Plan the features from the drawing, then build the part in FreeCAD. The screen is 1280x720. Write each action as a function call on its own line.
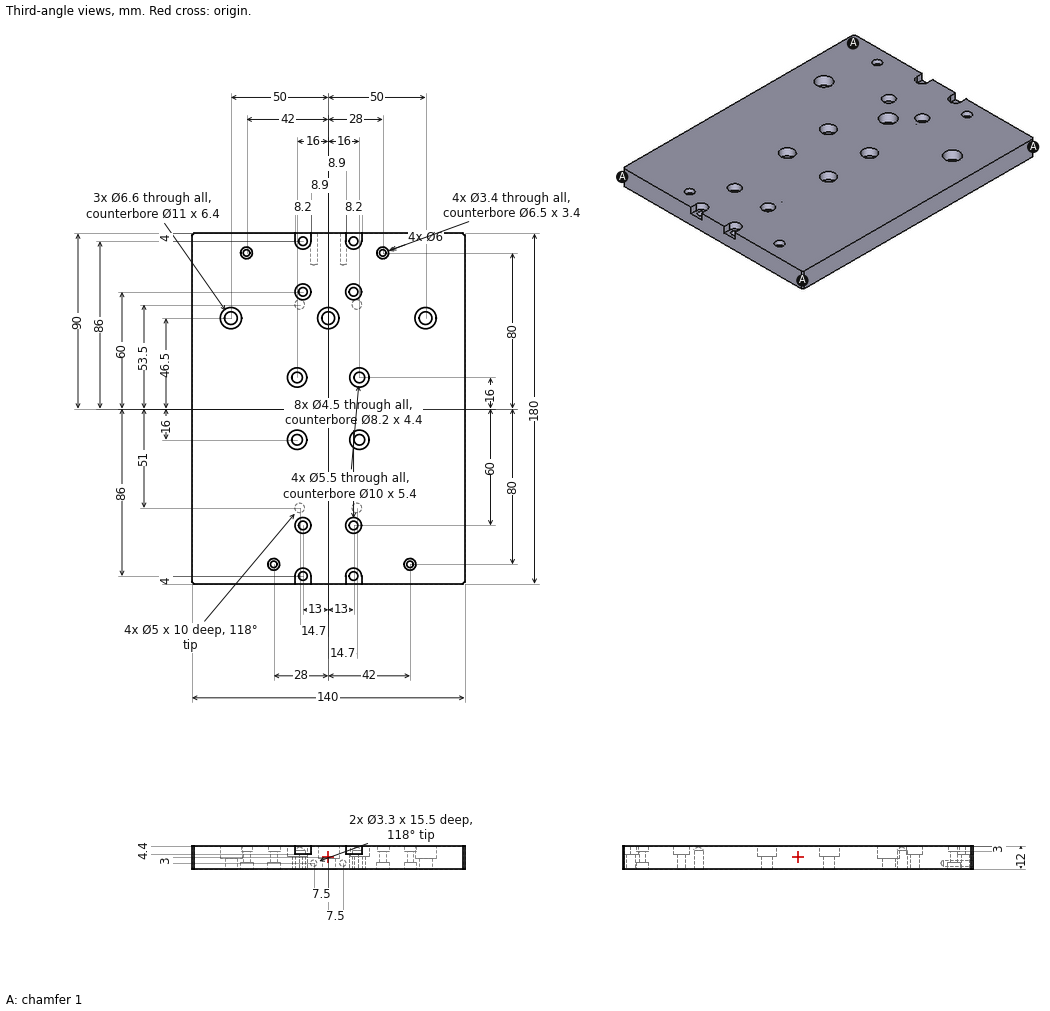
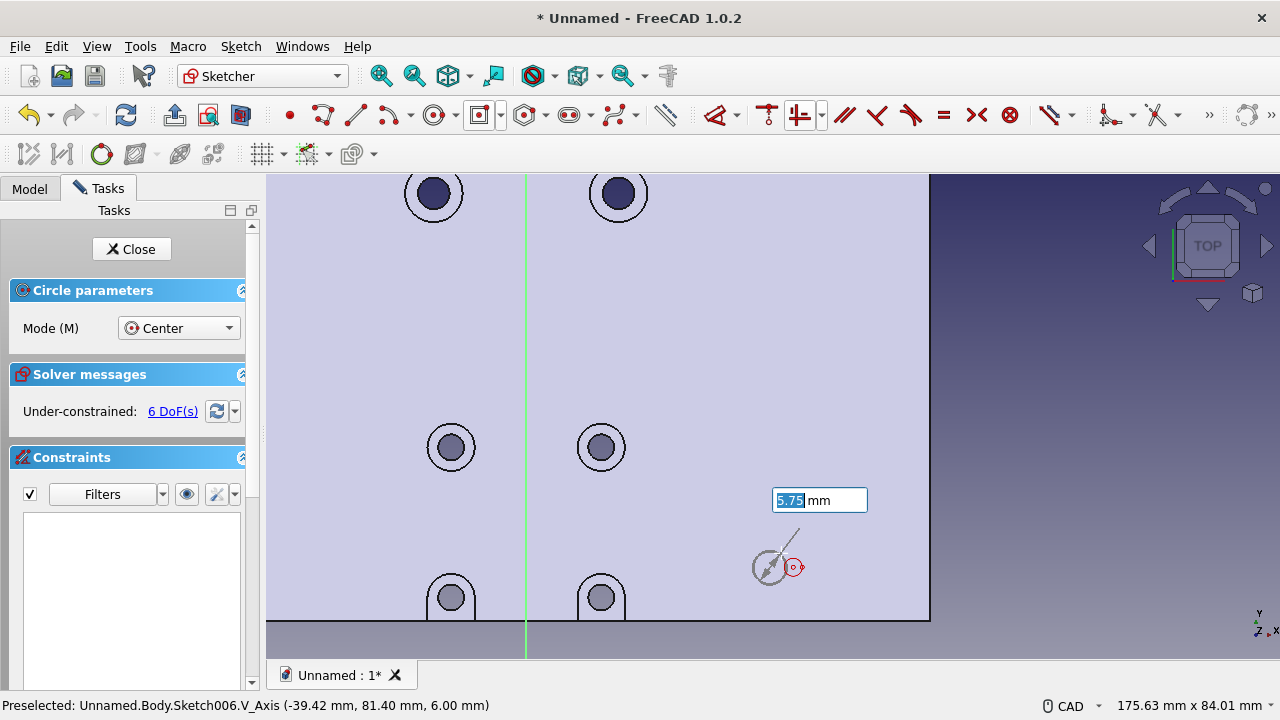
click(781, 551)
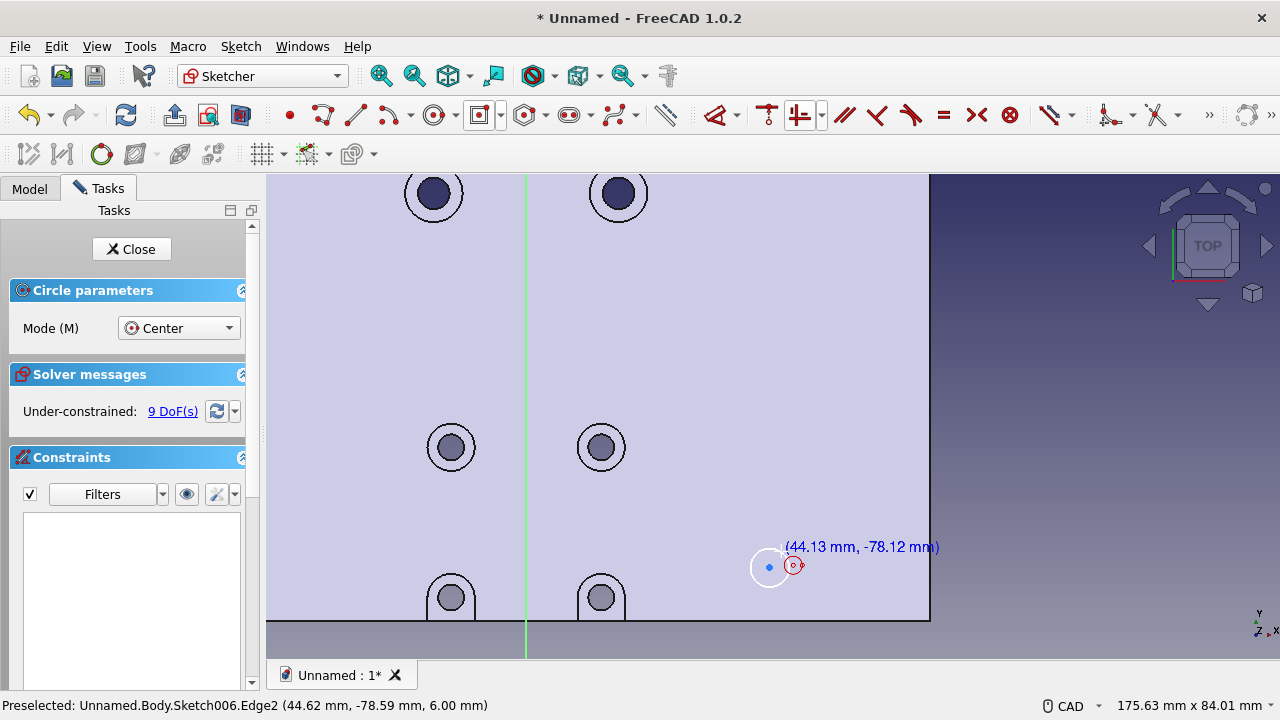
scroll(365, 563, up, 2)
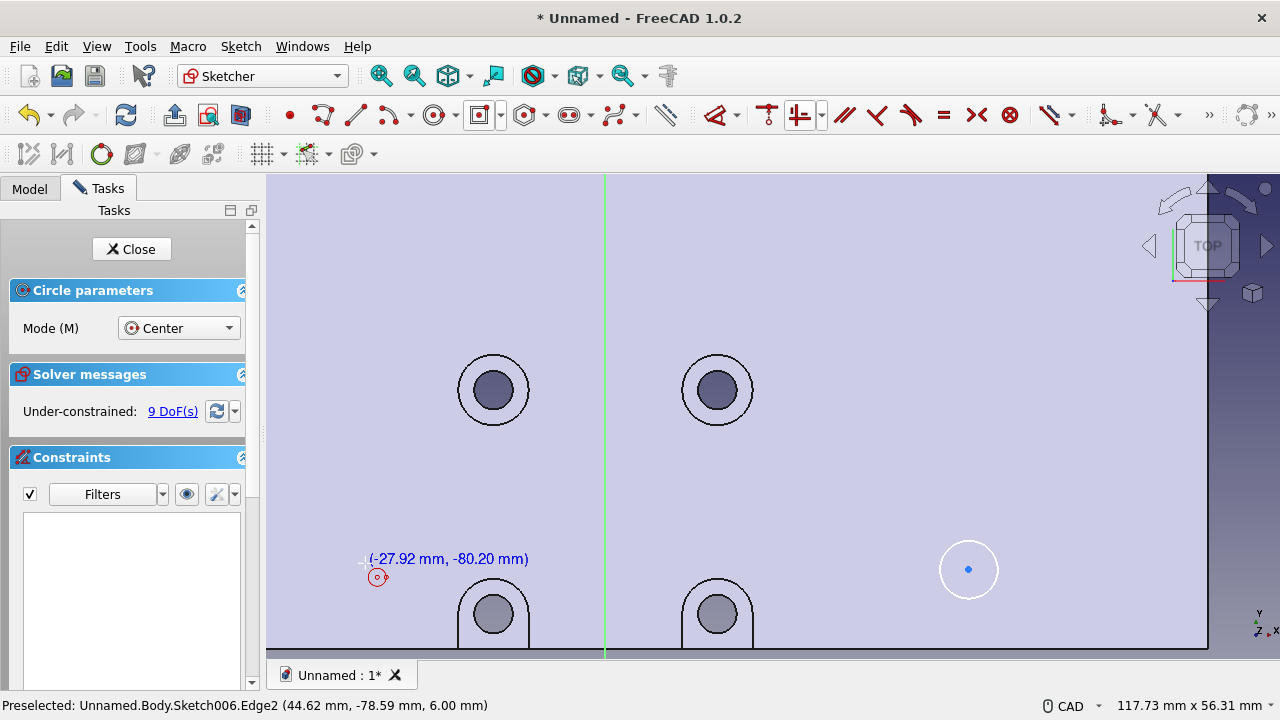
scroll(730, 554, down, 8)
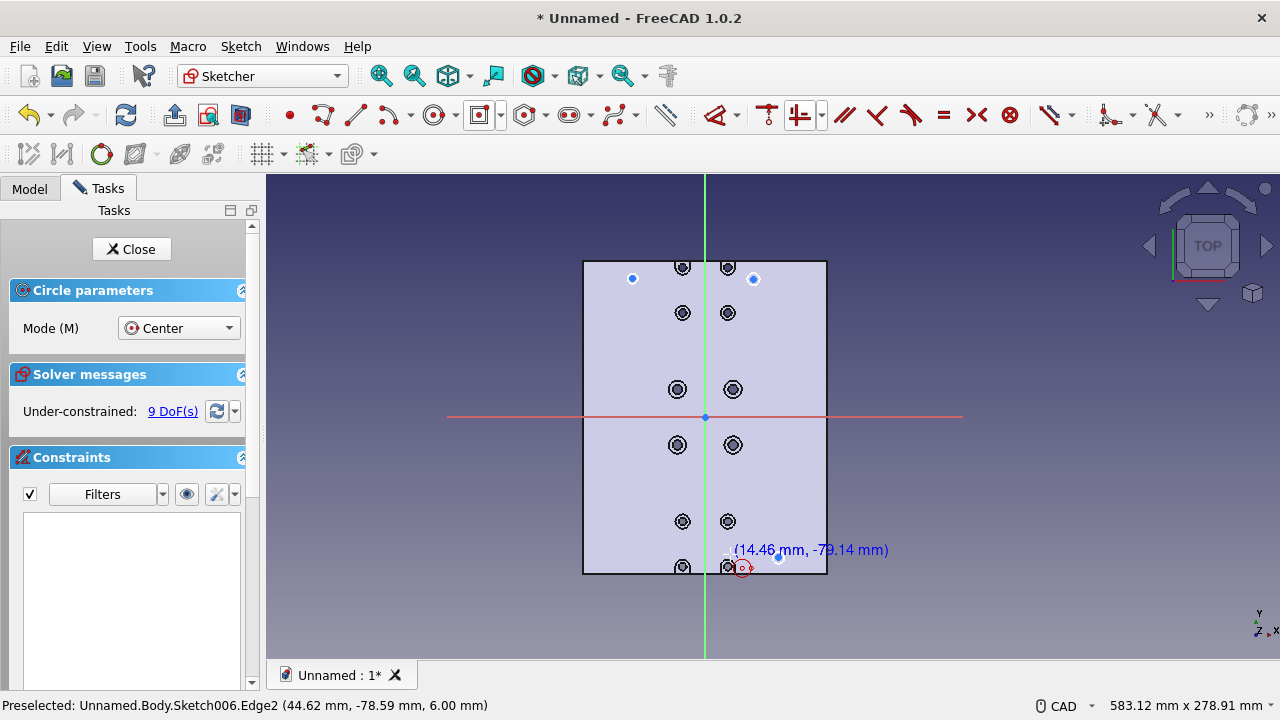
click(657, 556)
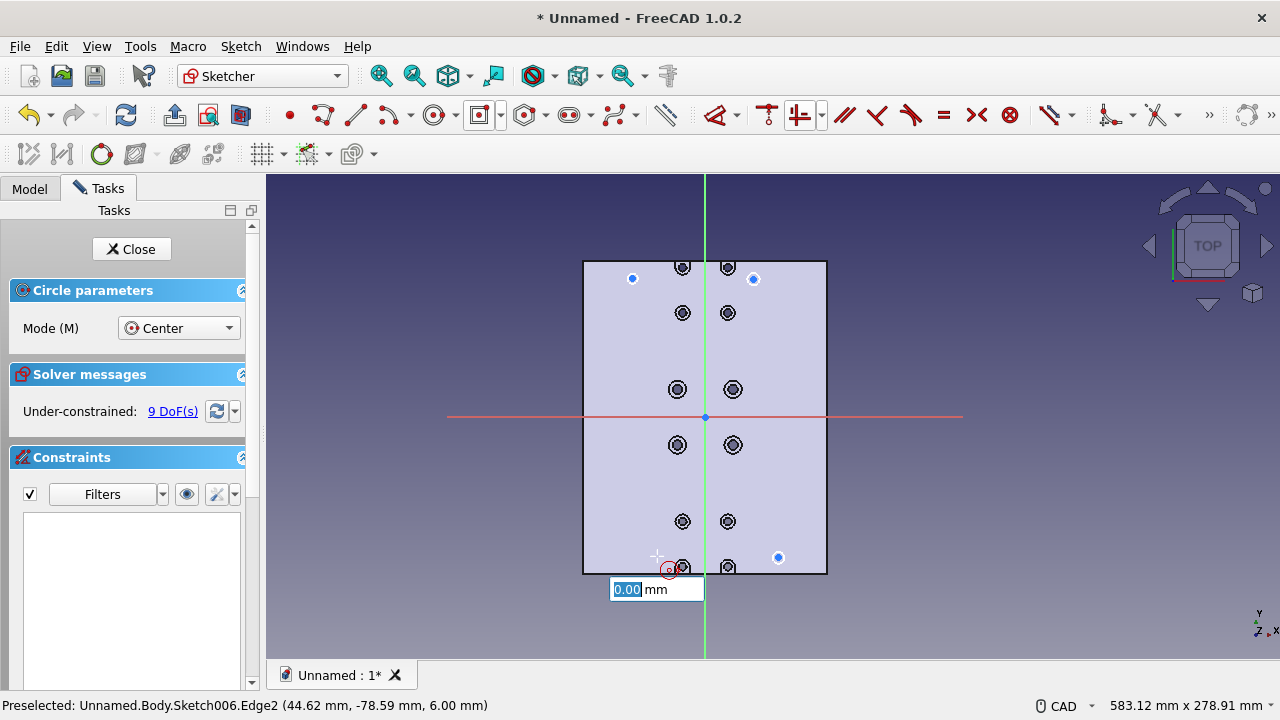
scroll(660, 553, up, 6)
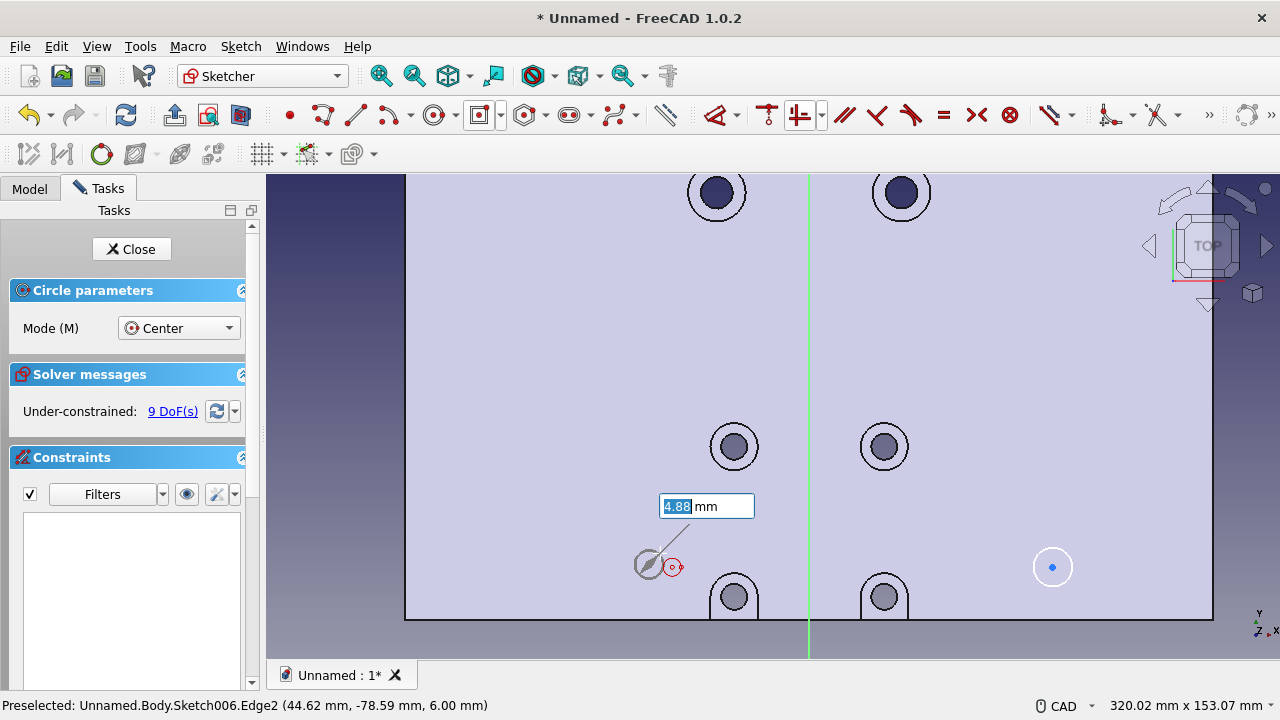
click(660, 550)
key(Escape)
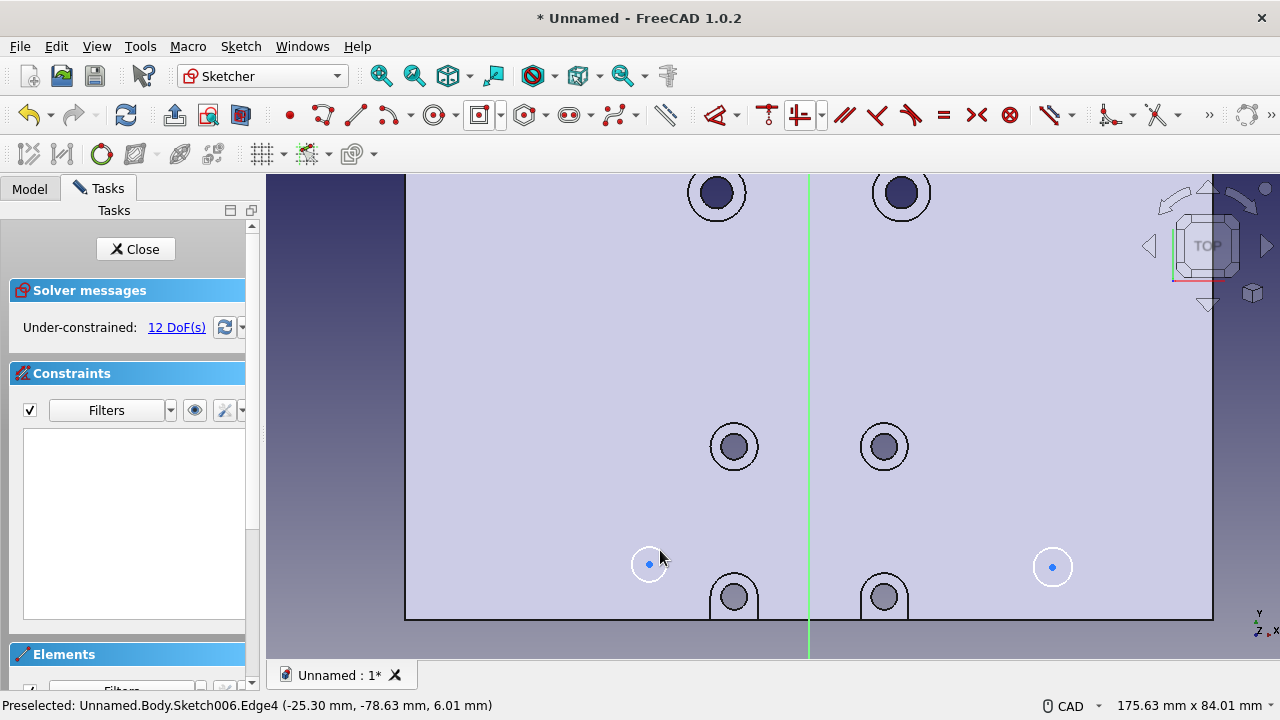
scroll(659, 553, down, 6)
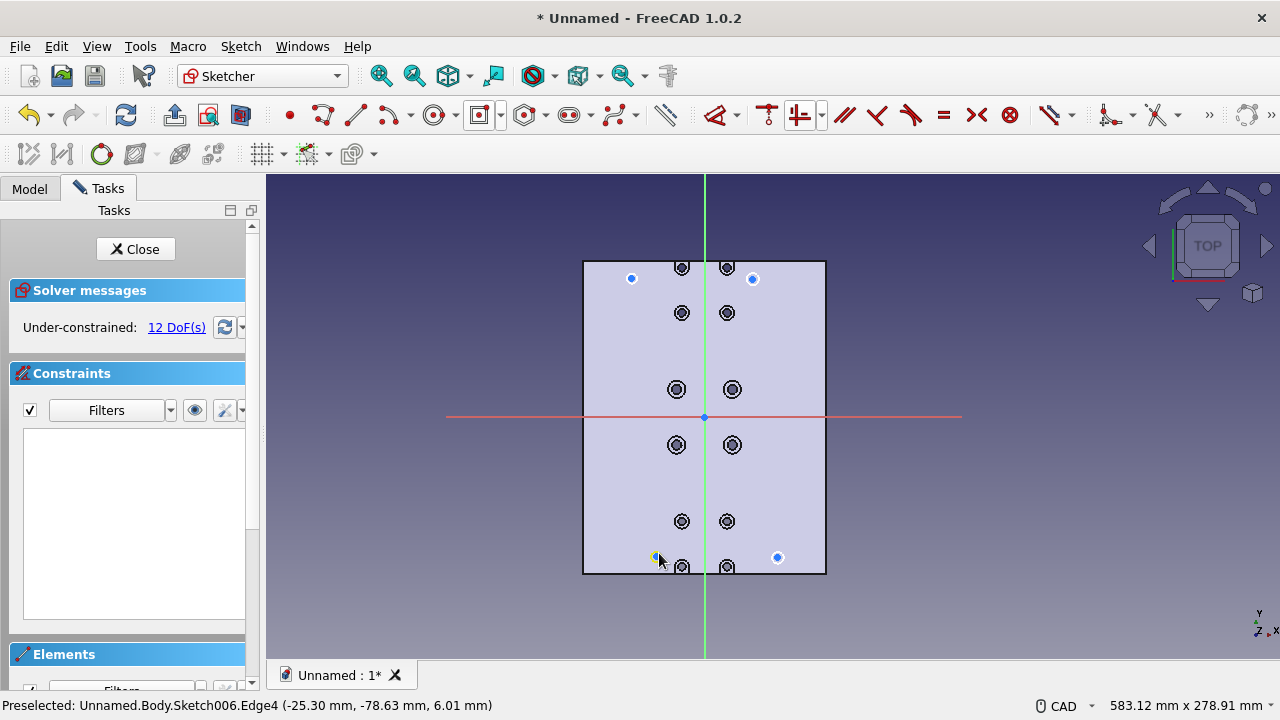
scroll(757, 275, up, 5)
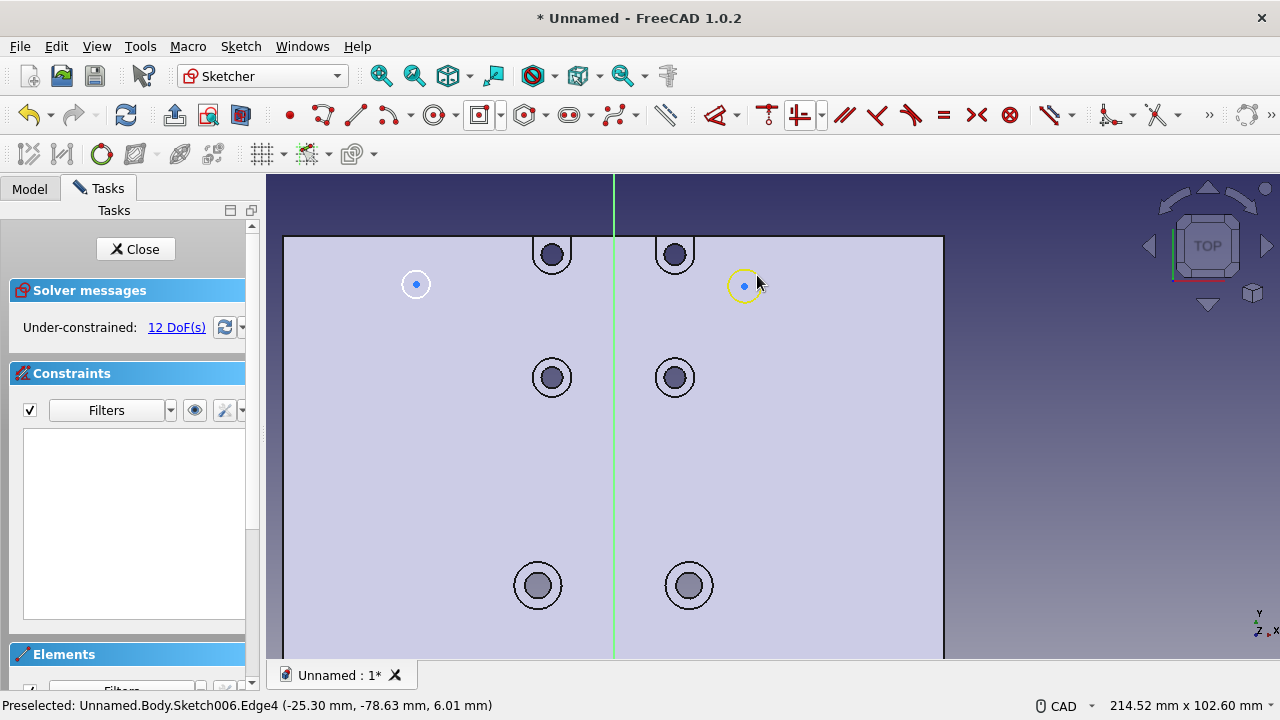
click(756, 274)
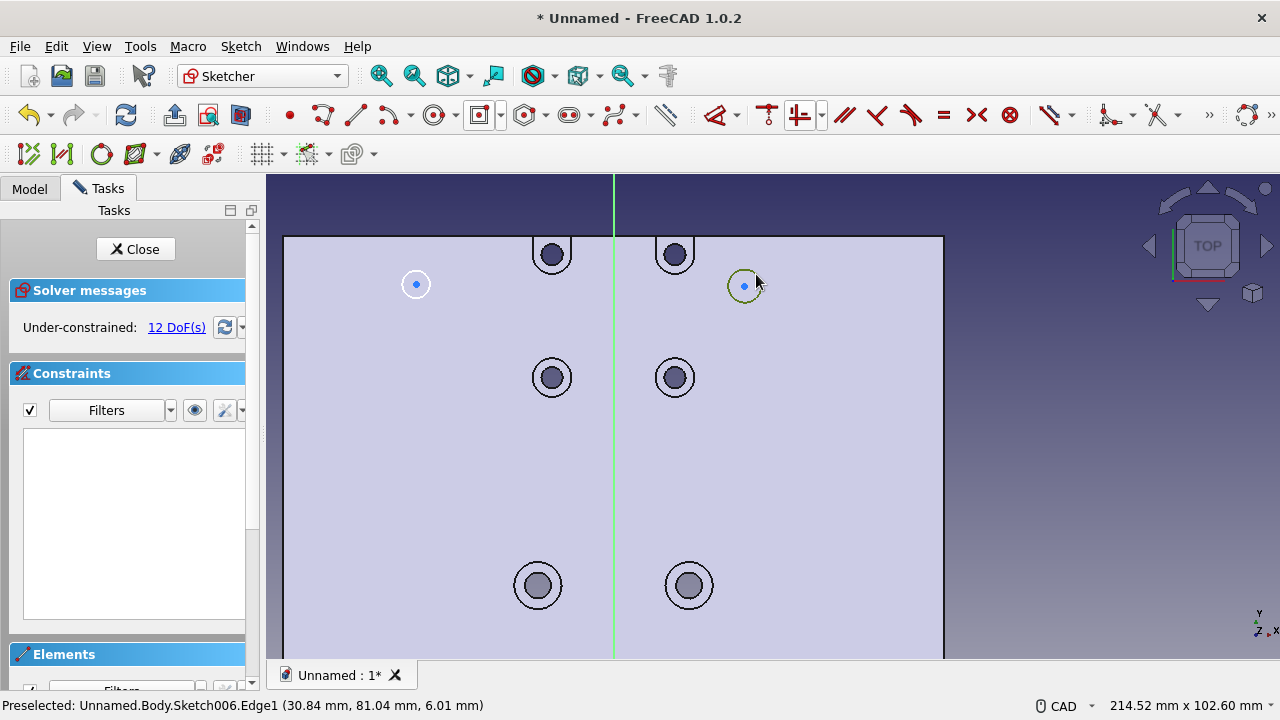
click(426, 275)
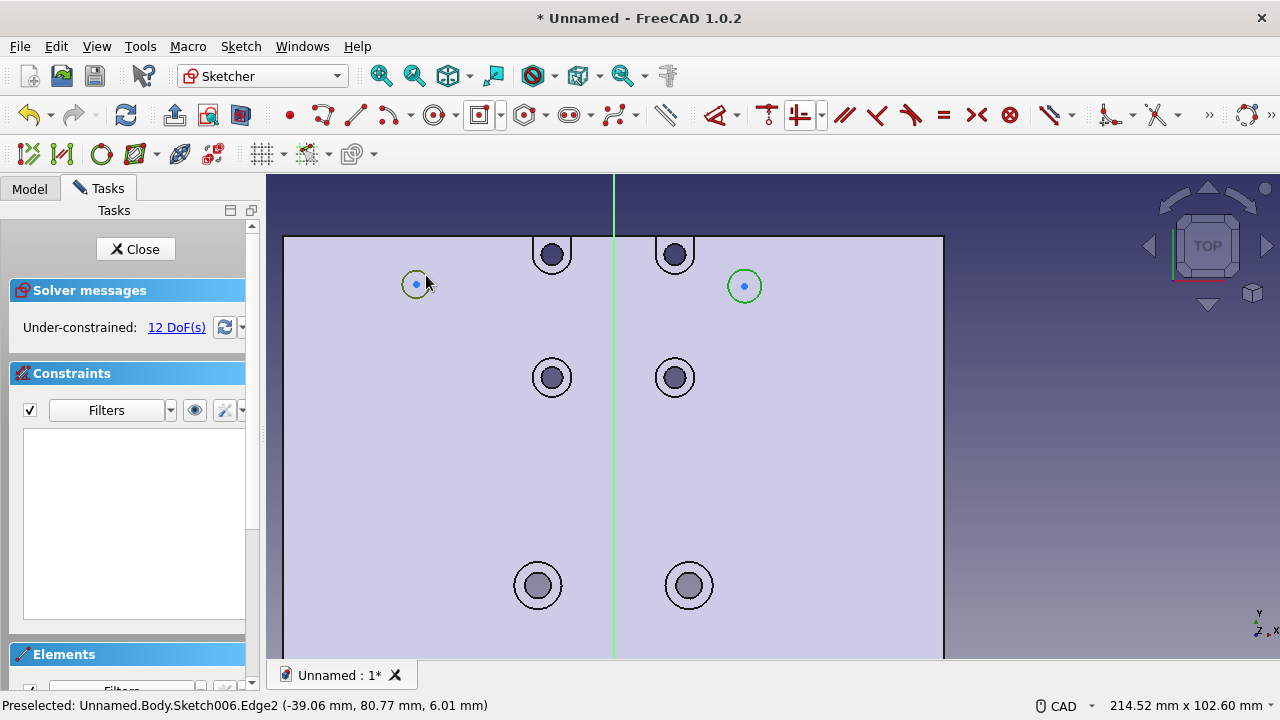
scroll(757, 274, down, 5)